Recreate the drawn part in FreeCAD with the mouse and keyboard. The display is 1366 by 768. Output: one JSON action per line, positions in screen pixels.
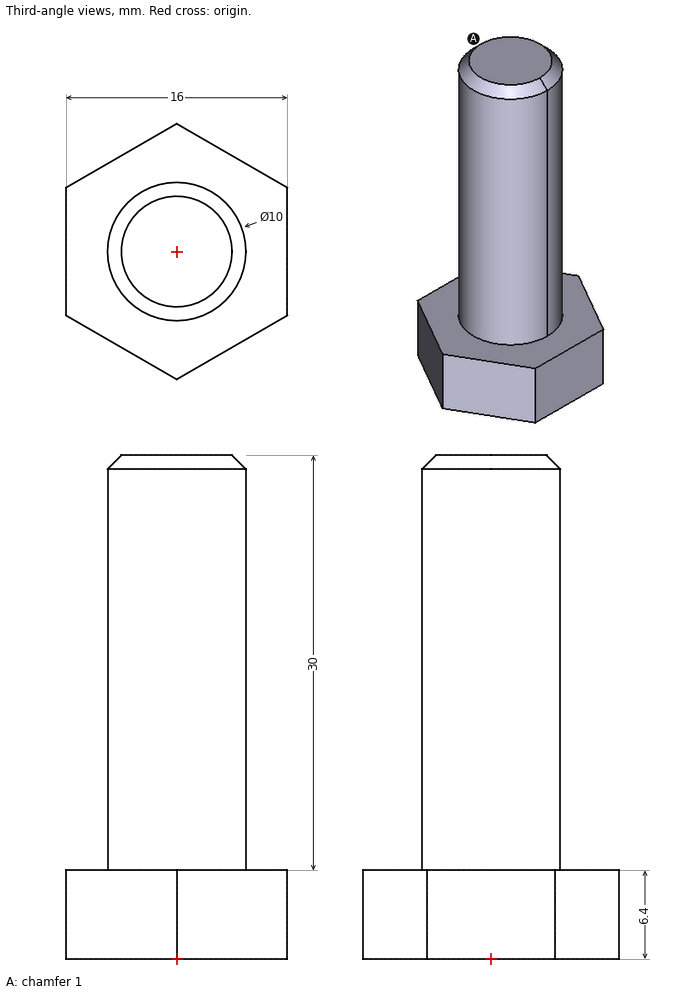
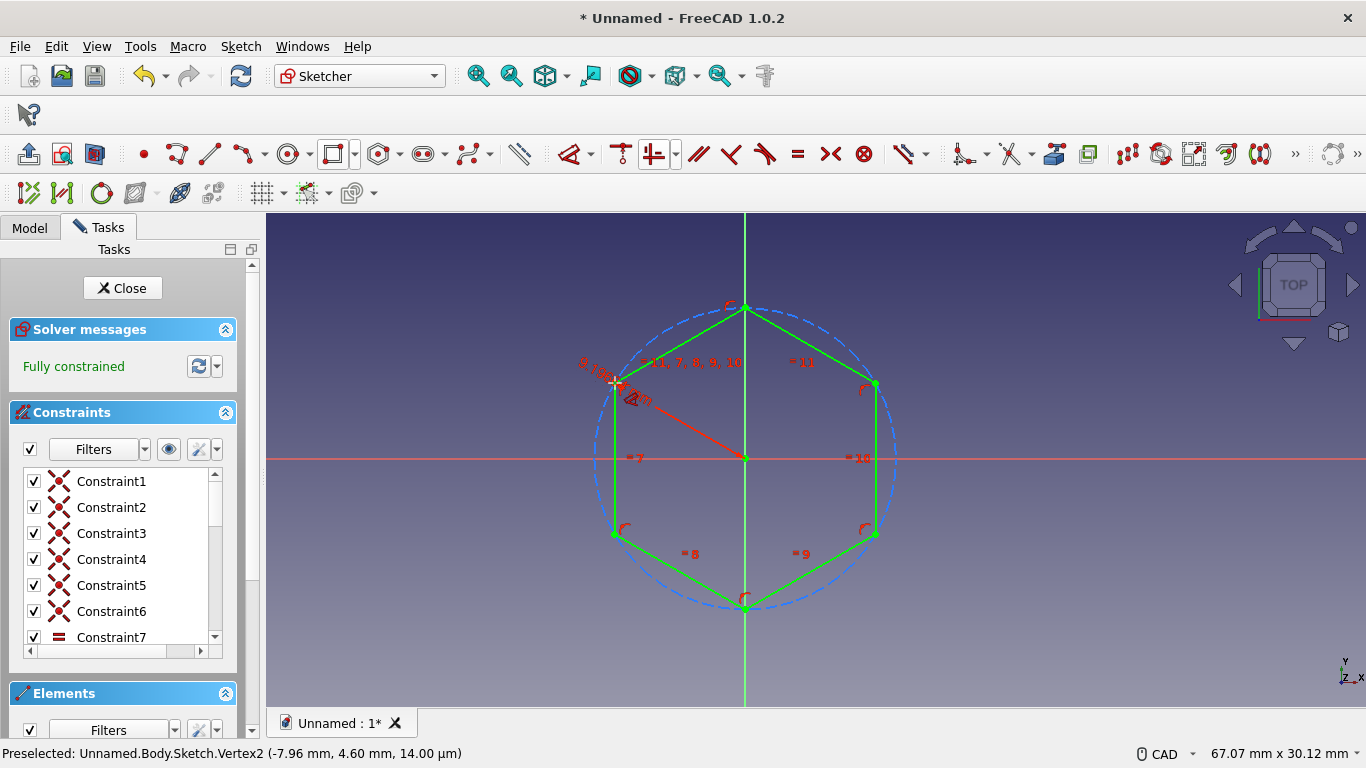
{"action": "left_click", "coordinate": [876, 534]}
{"action": "left_click", "coordinate": [685, 616]}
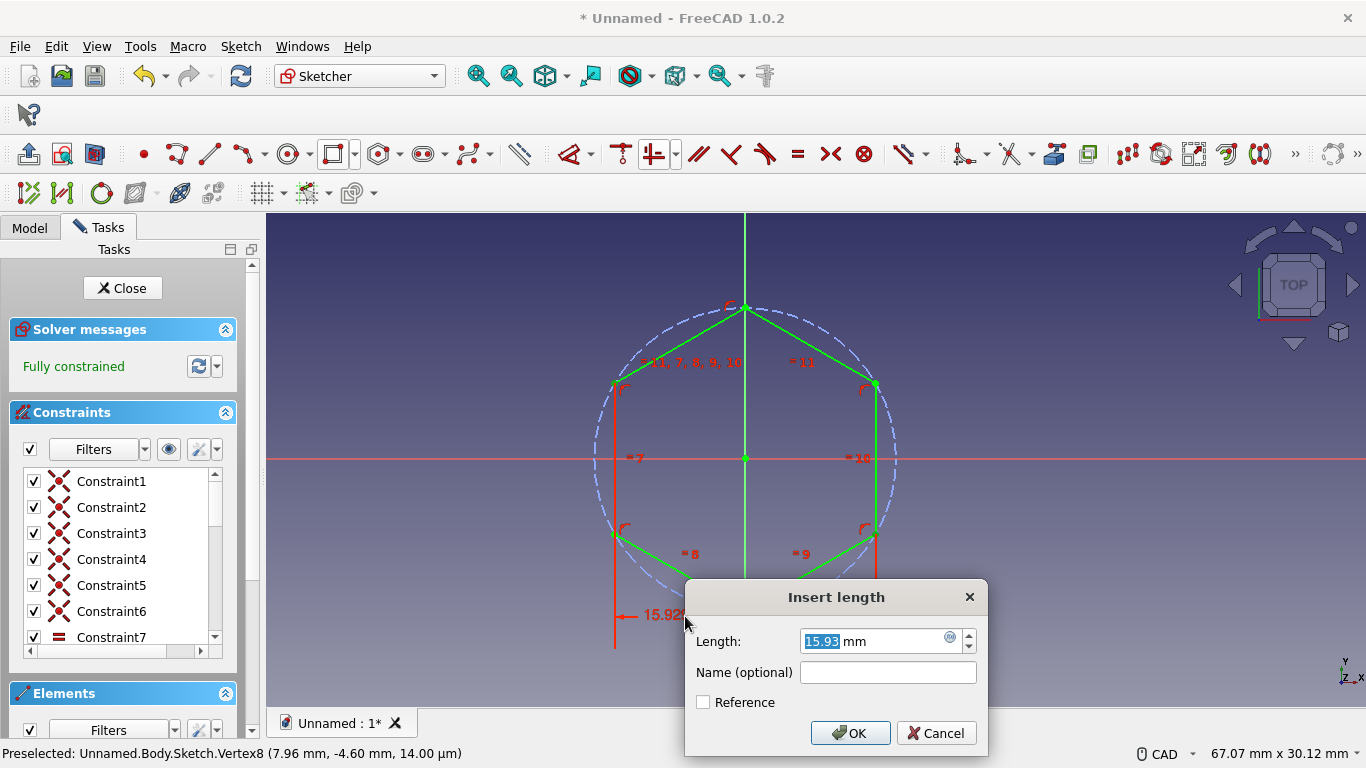
{"action": "type", "text": "16"}
{"action": "key", "text": "Return"}
{"action": "key", "text": "Escape"}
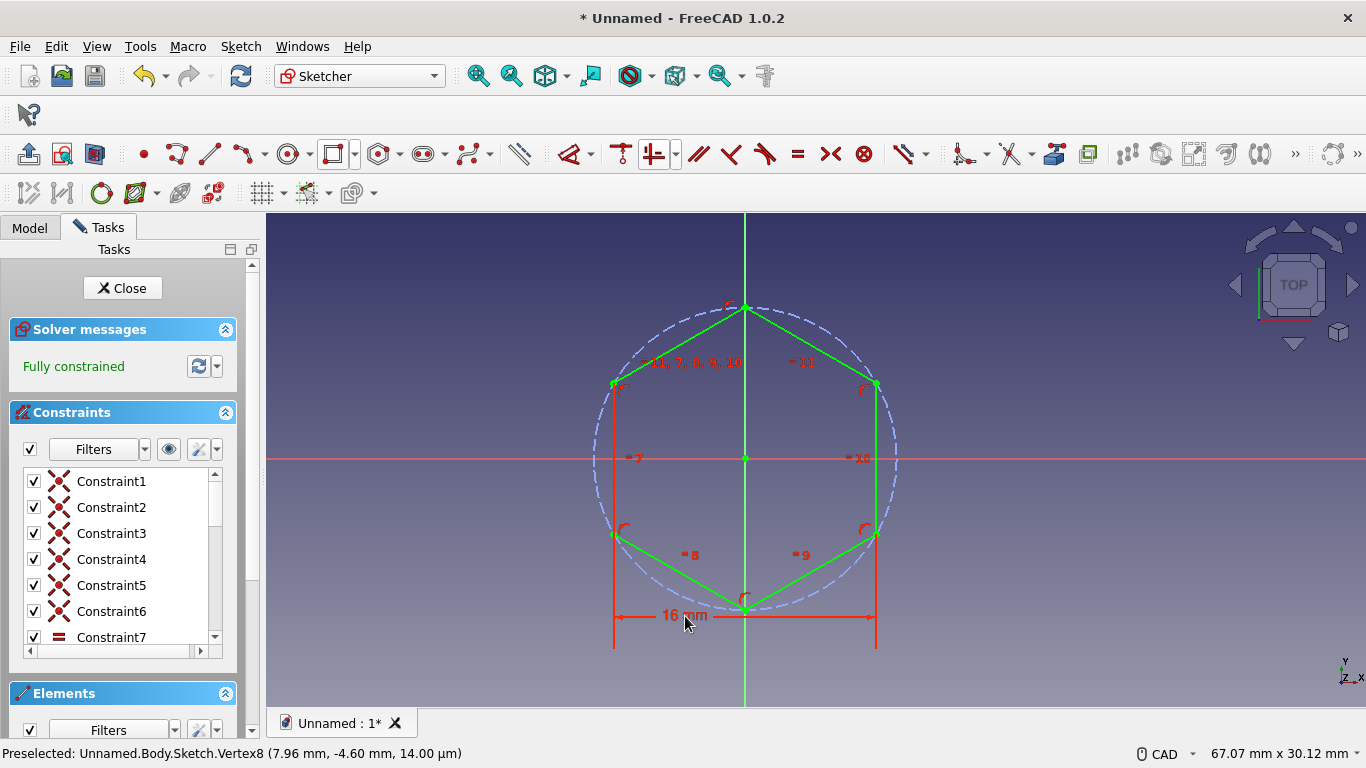
{"action": "left_click", "coordinate": [123, 288]}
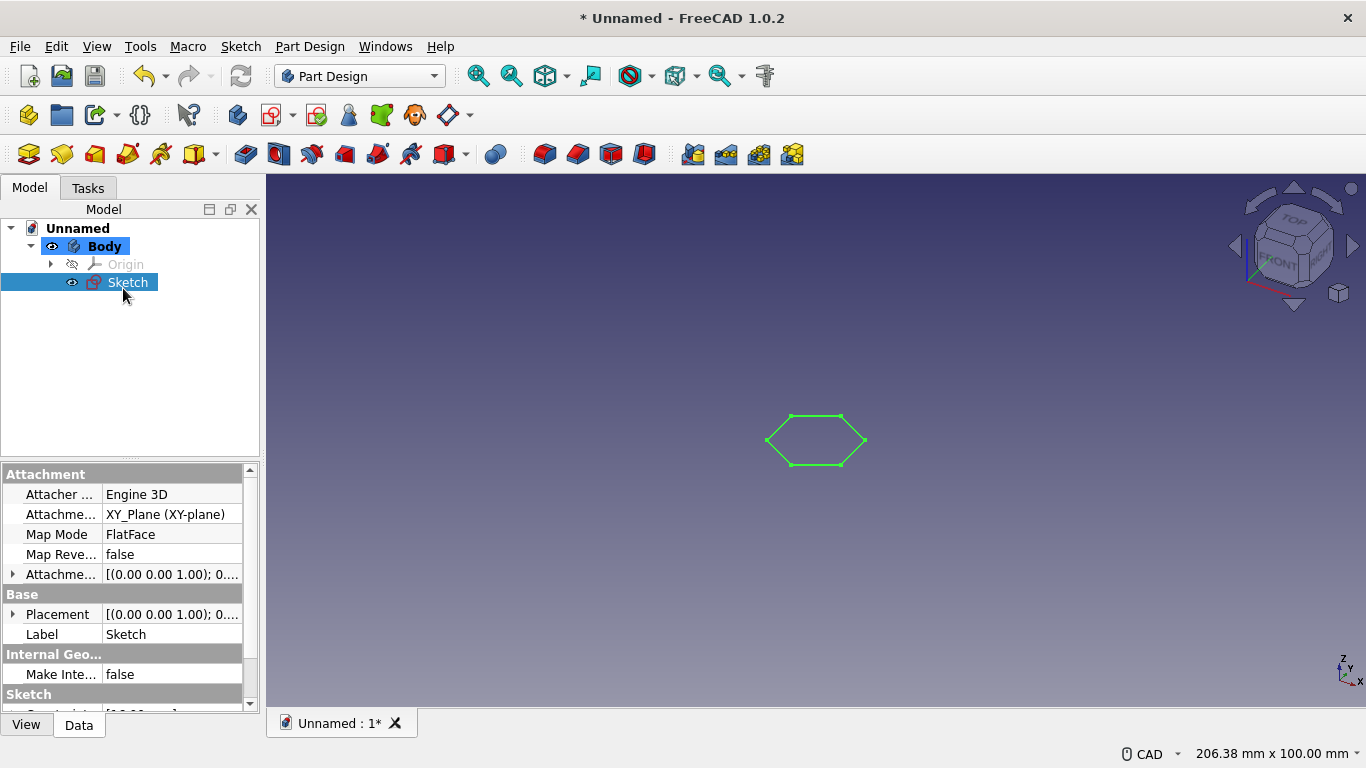
{"action": "left_click", "coordinate": [29, 154]}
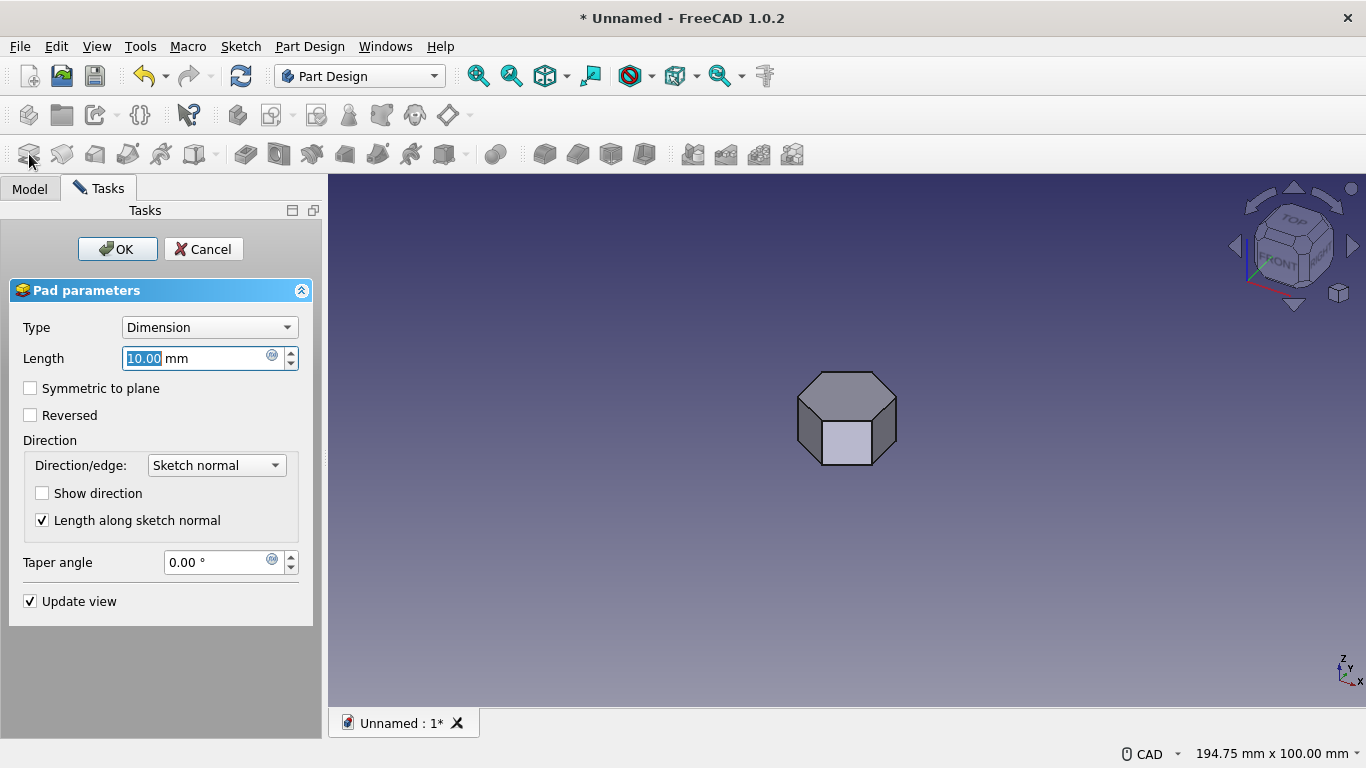
{"action": "type", "text": "6.4"}
{"action": "key", "text": "Tab"}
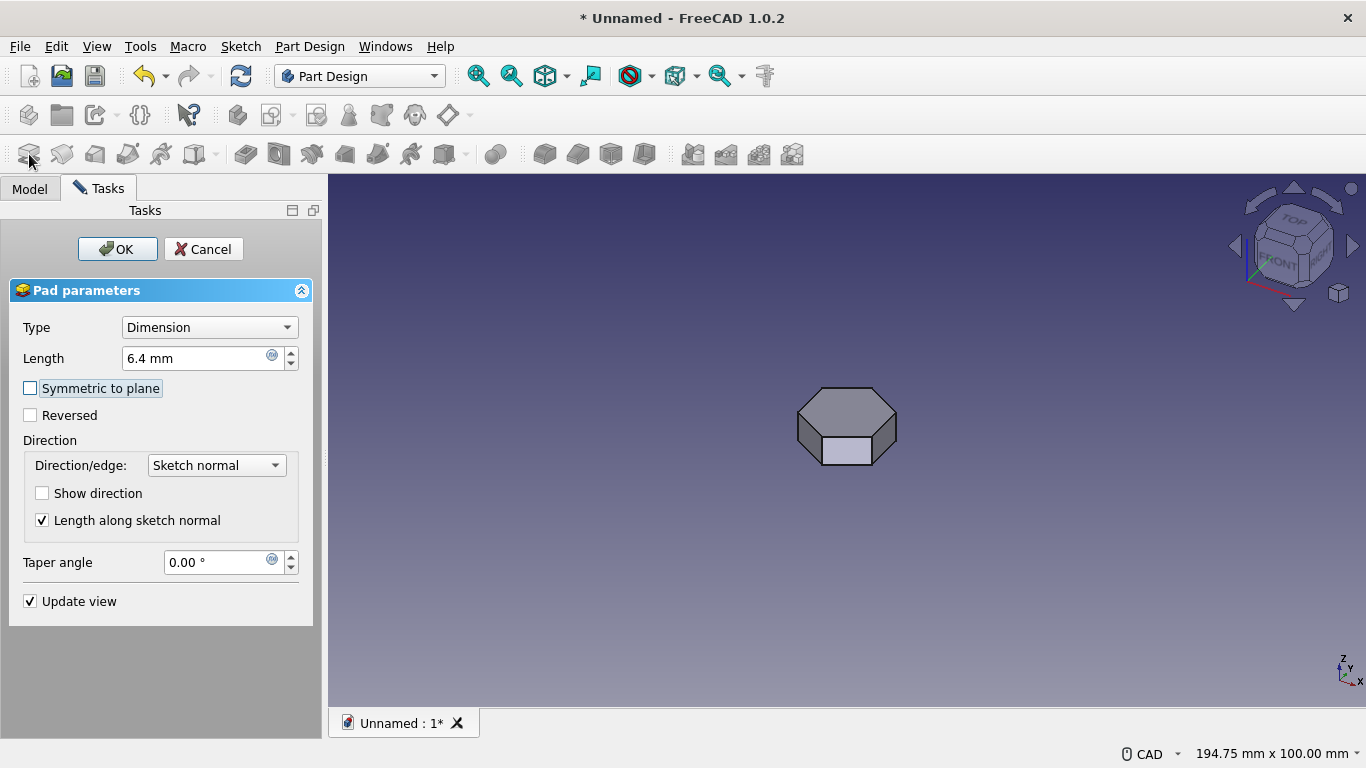
{"action": "left_click", "coordinate": [118, 249]}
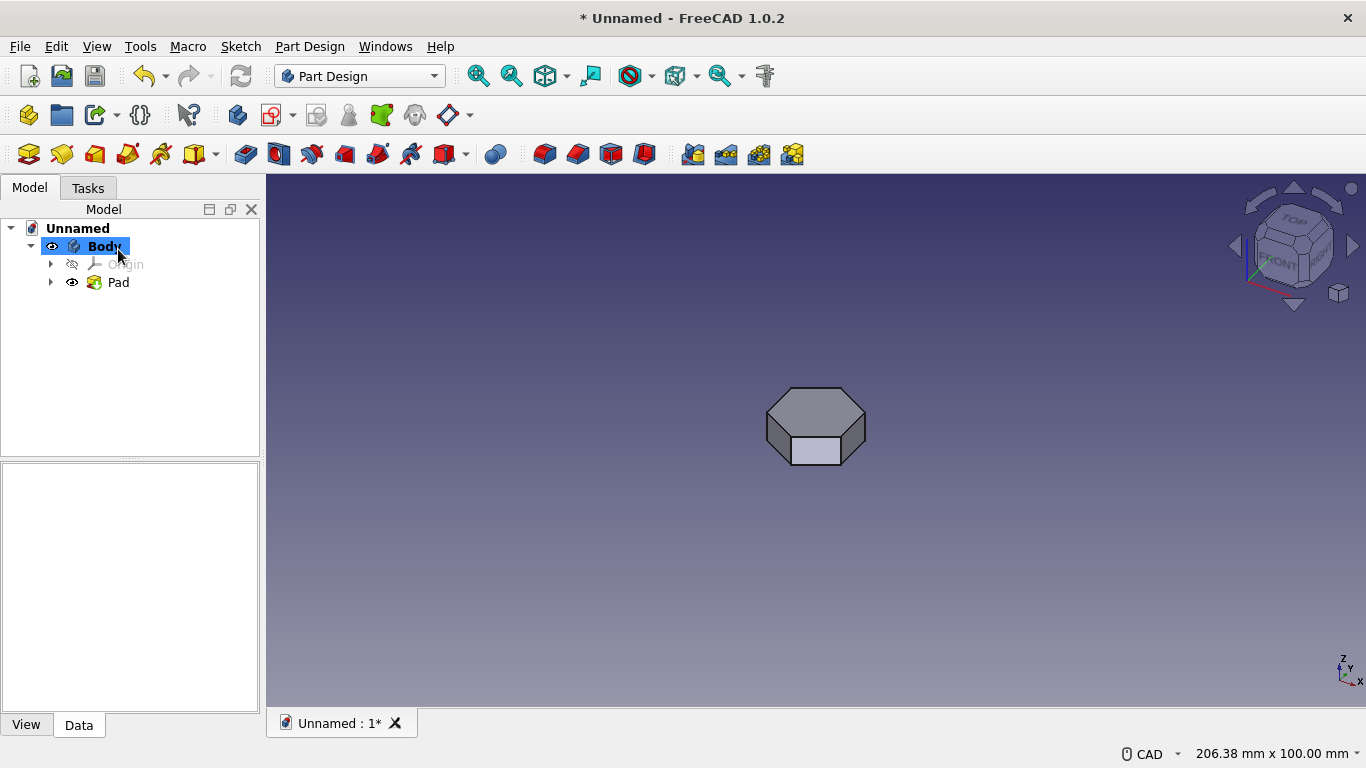
{"action": "left_click", "coordinate": [479, 76]}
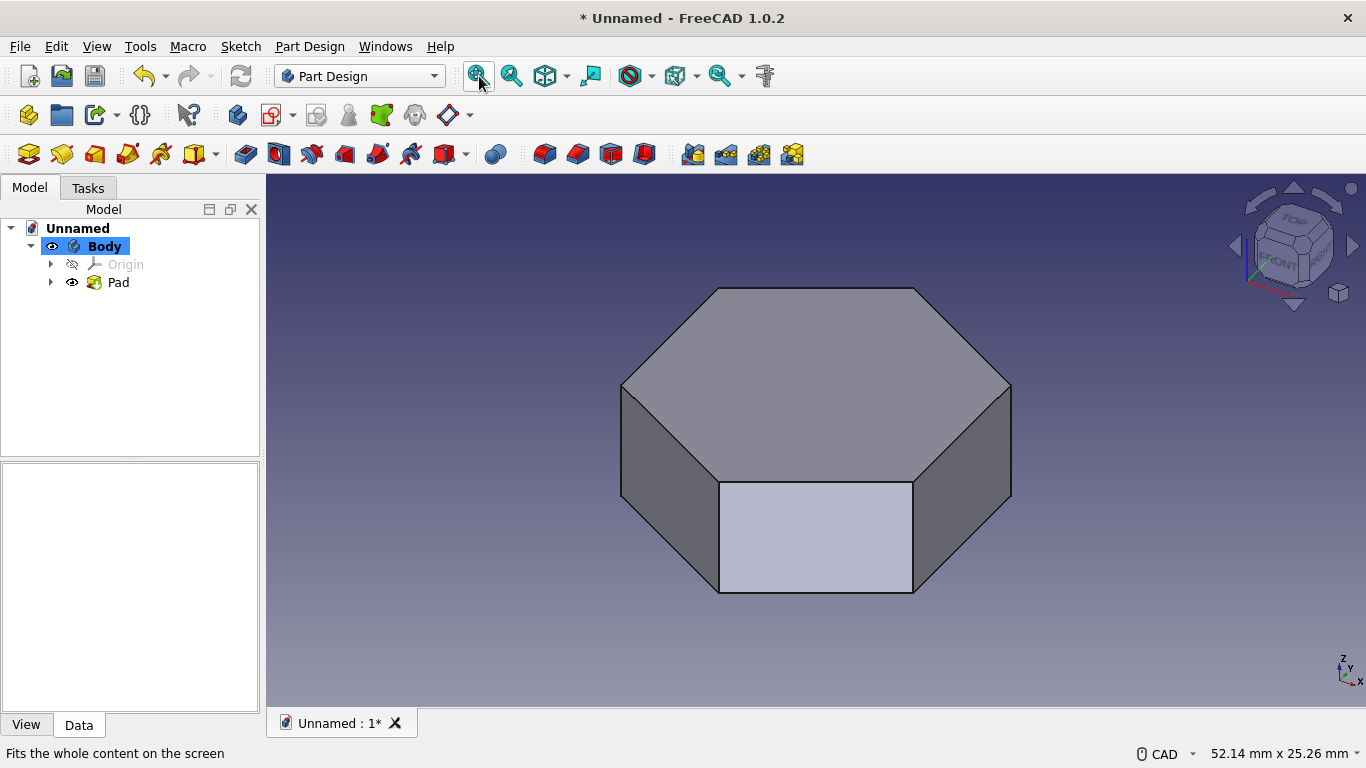
{"action": "left_click", "coordinate": [816, 384]}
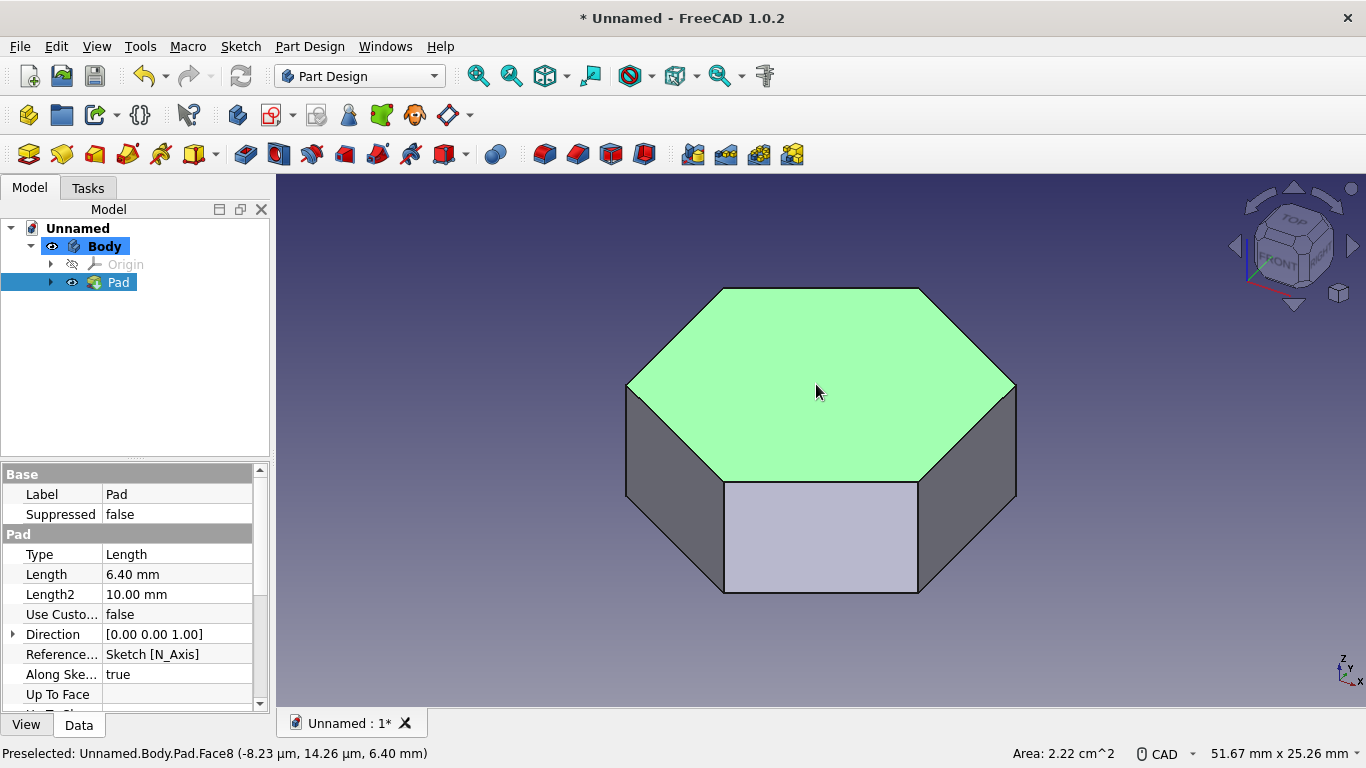
{"action": "left_click", "coordinate": [270, 116]}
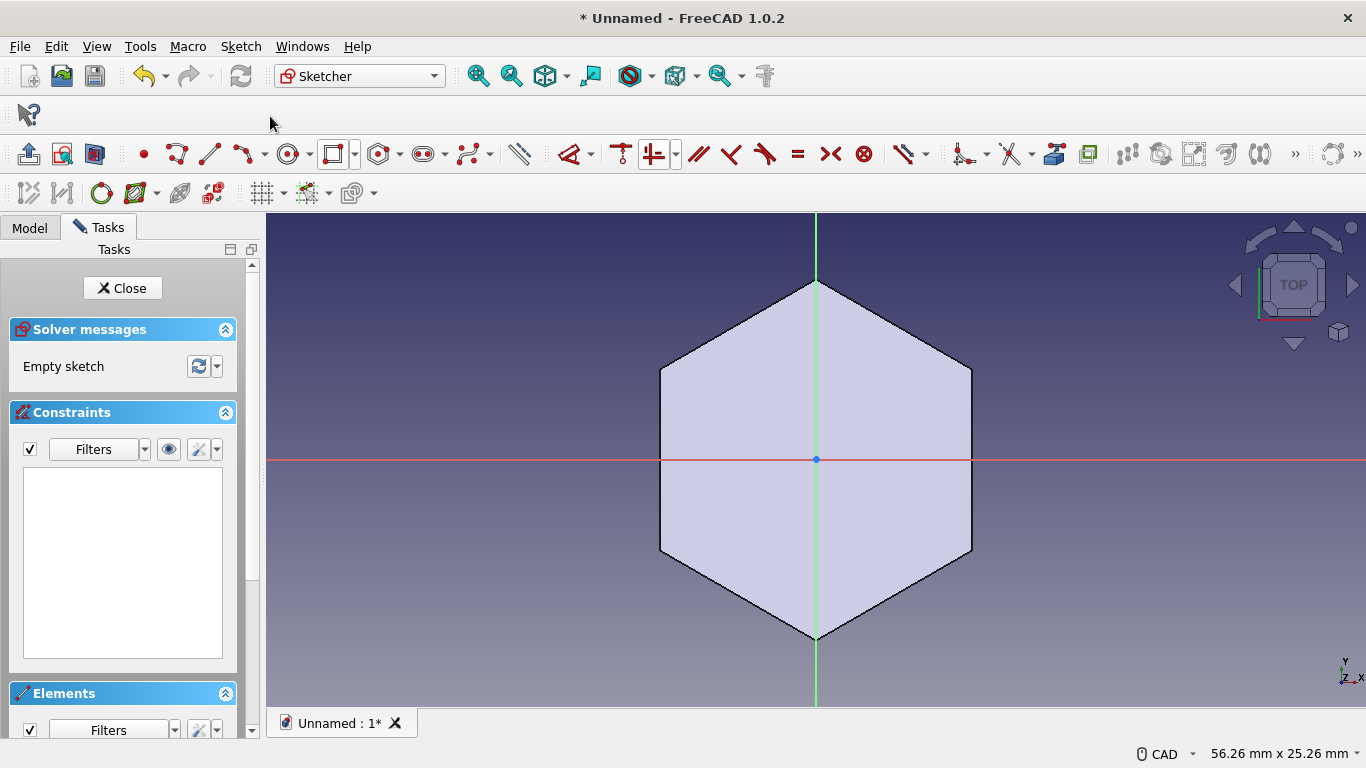
{"action": "scroll", "coordinate": [955, 460], "scroll_direction": "up", "scroll_amount": 2}